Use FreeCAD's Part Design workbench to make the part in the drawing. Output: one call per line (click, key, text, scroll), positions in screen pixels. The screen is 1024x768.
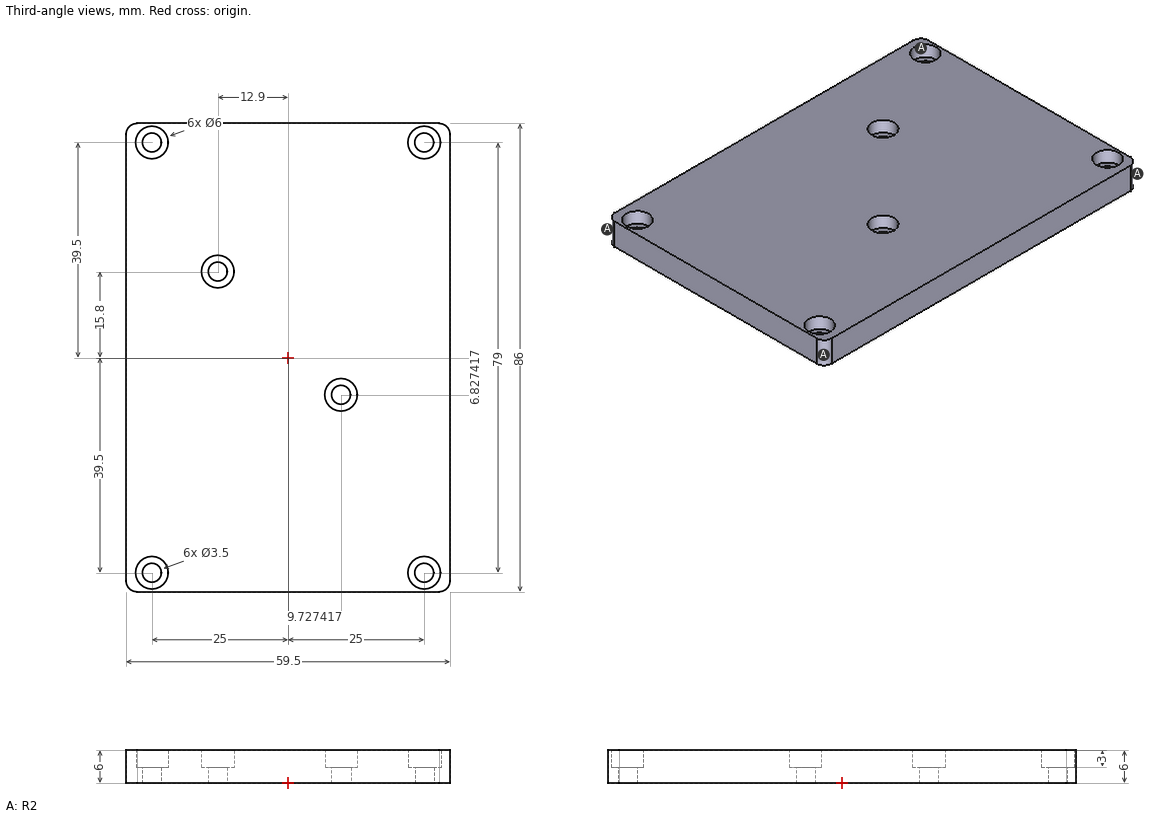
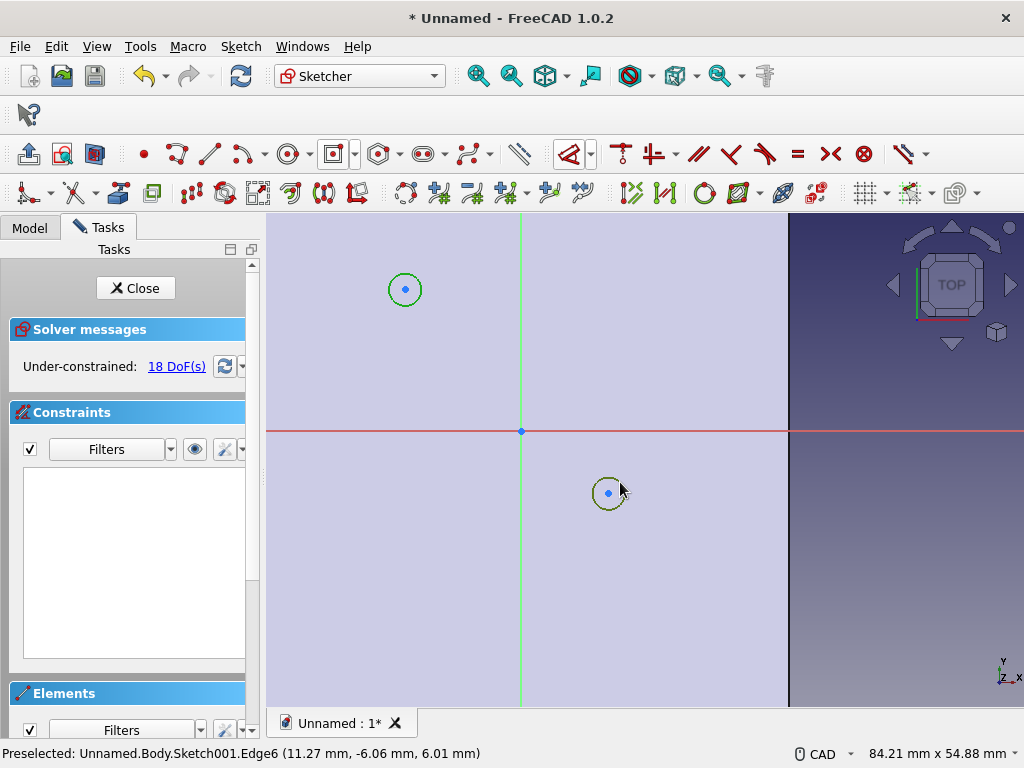
key(e)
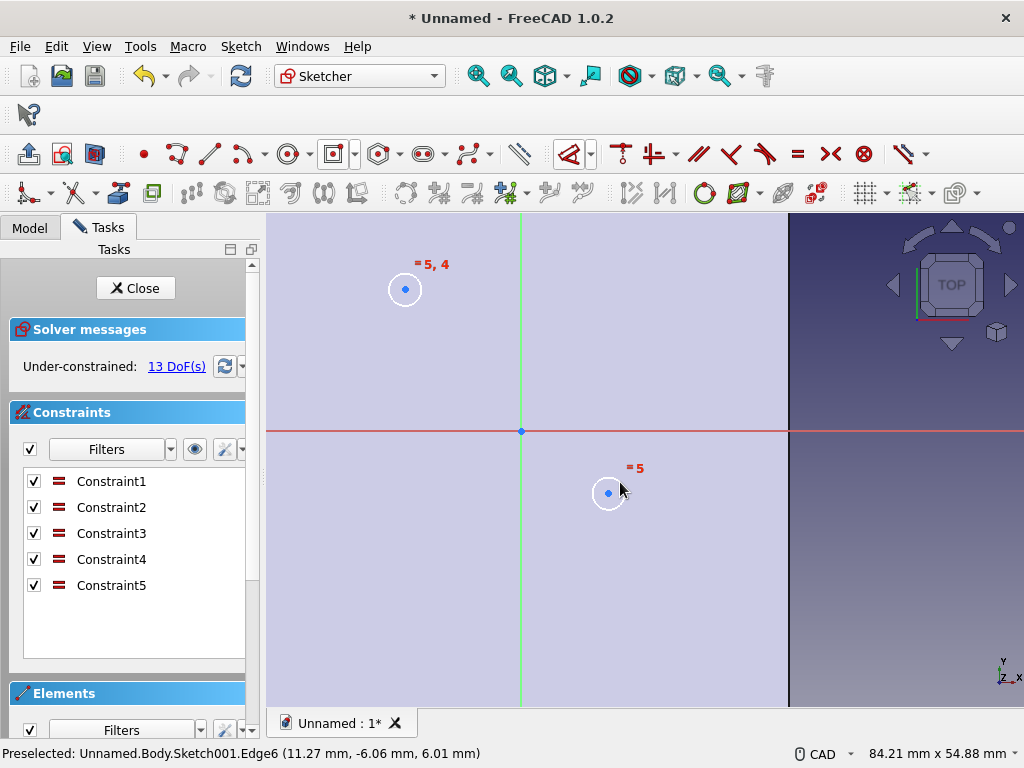
scroll(621, 483, down, 4)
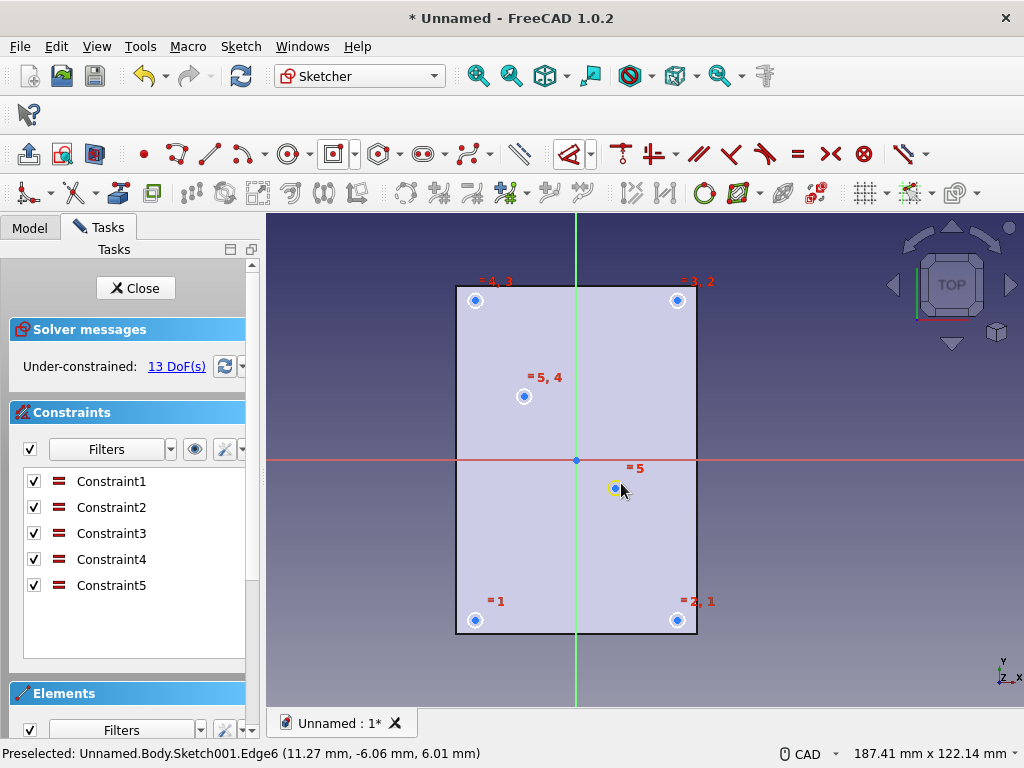
click(475, 620)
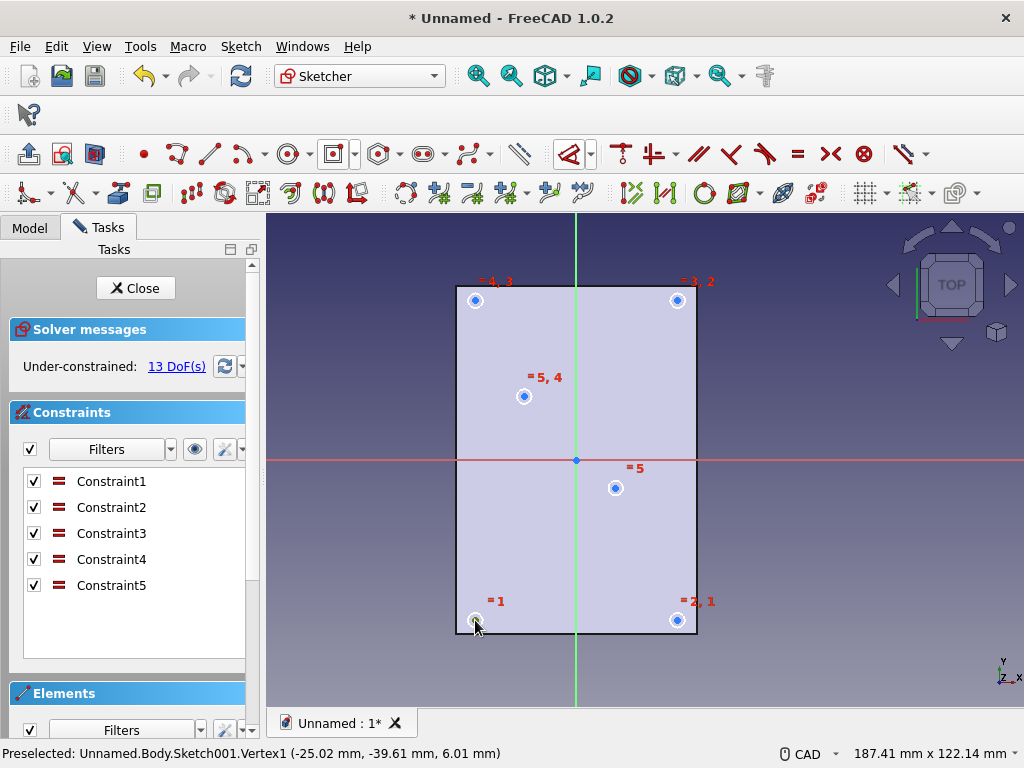
click(677, 620)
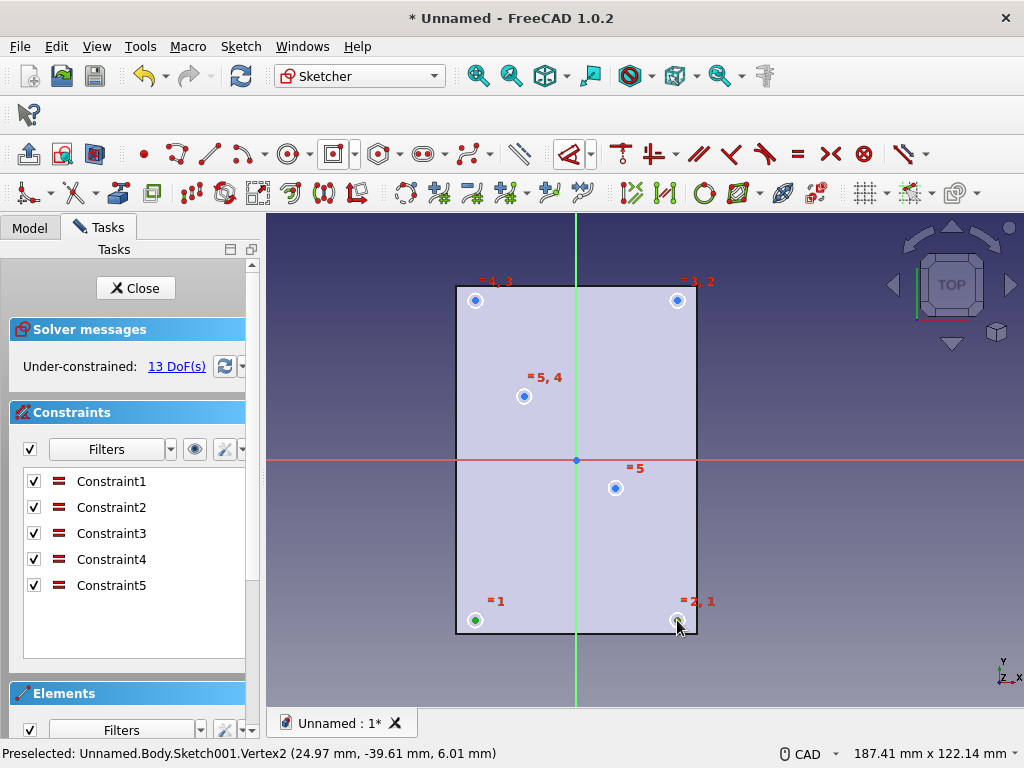
key(h)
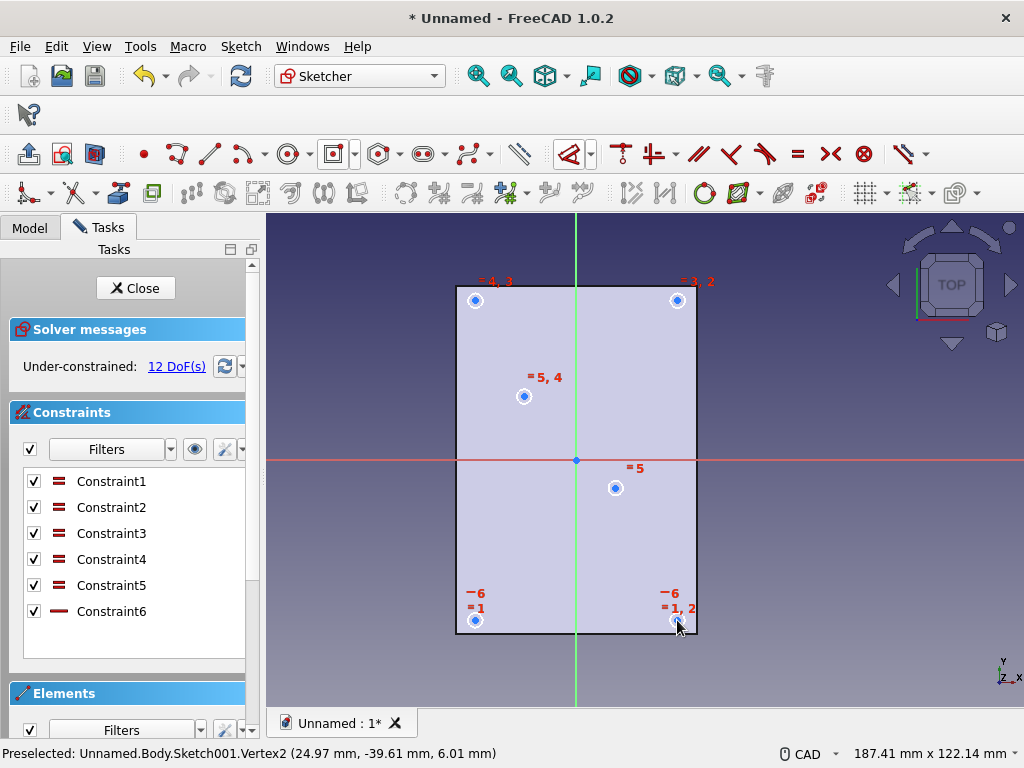
click(677, 620)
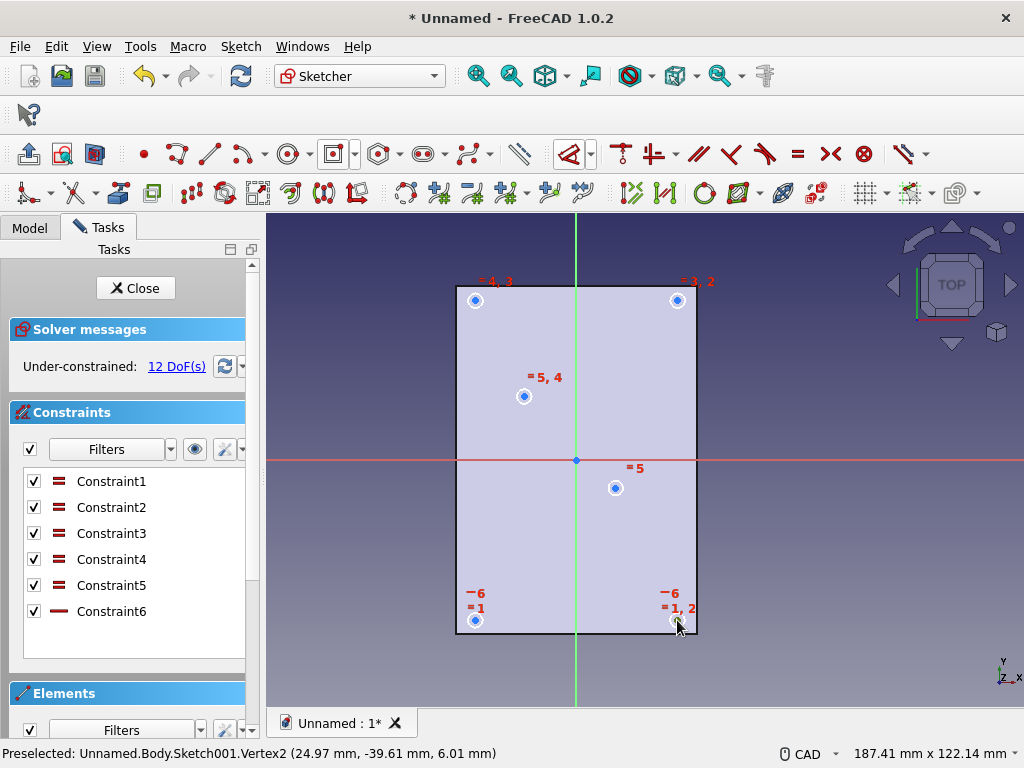
click(678, 301)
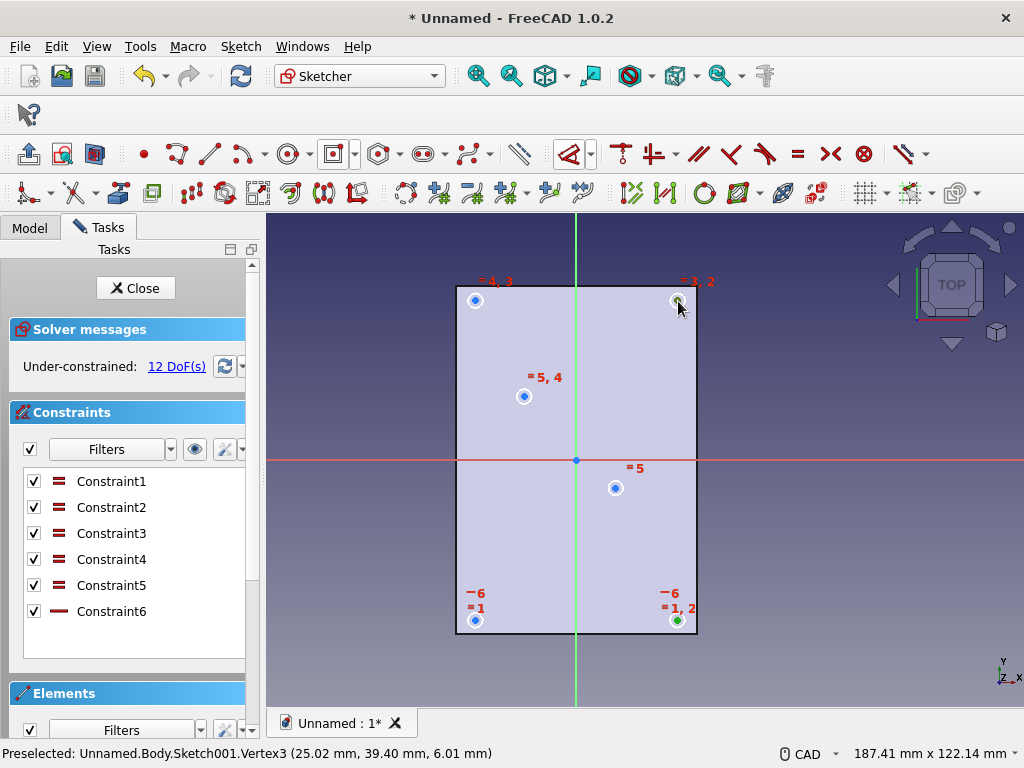
key(v)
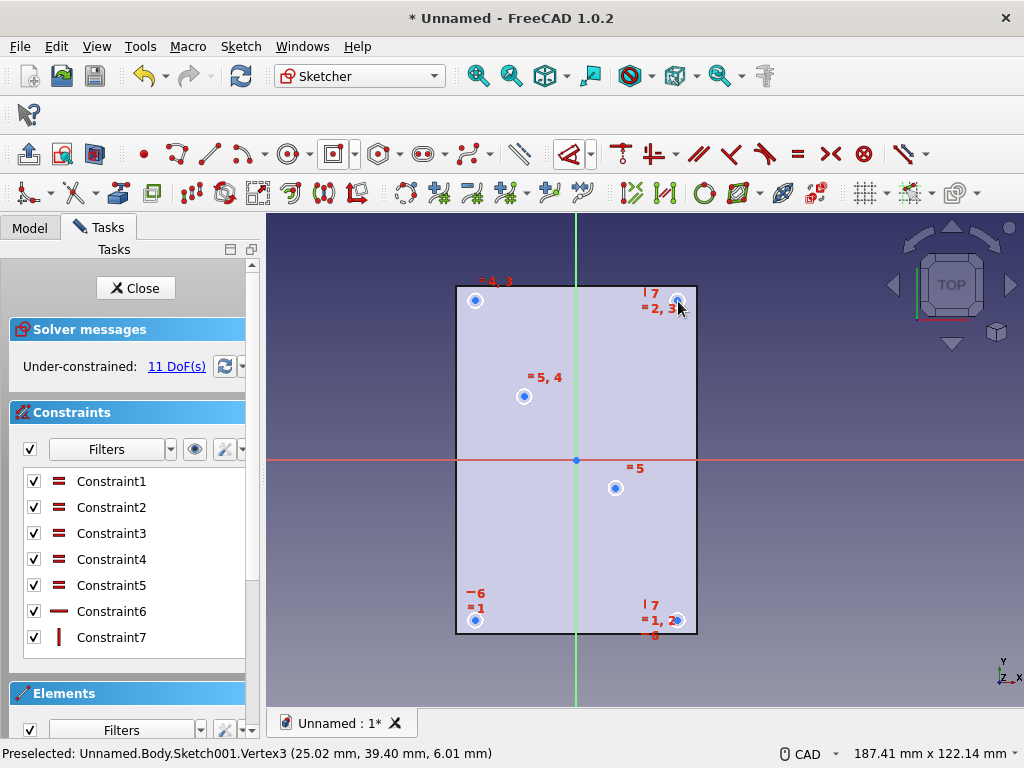
click(475, 620)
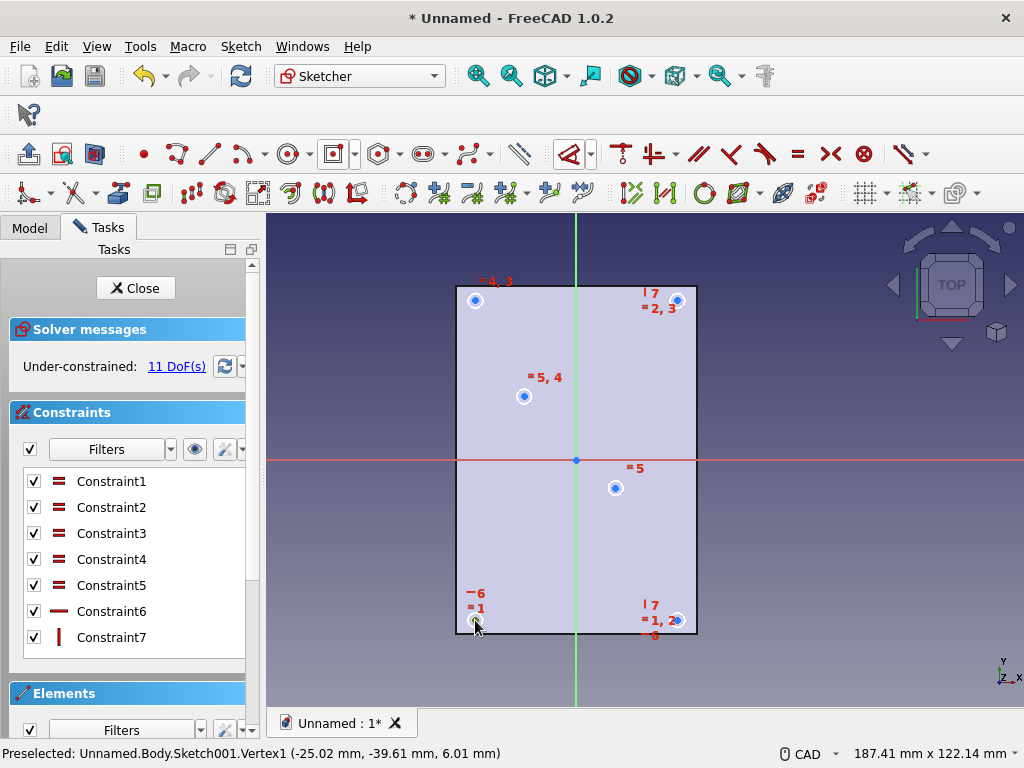
click(475, 301)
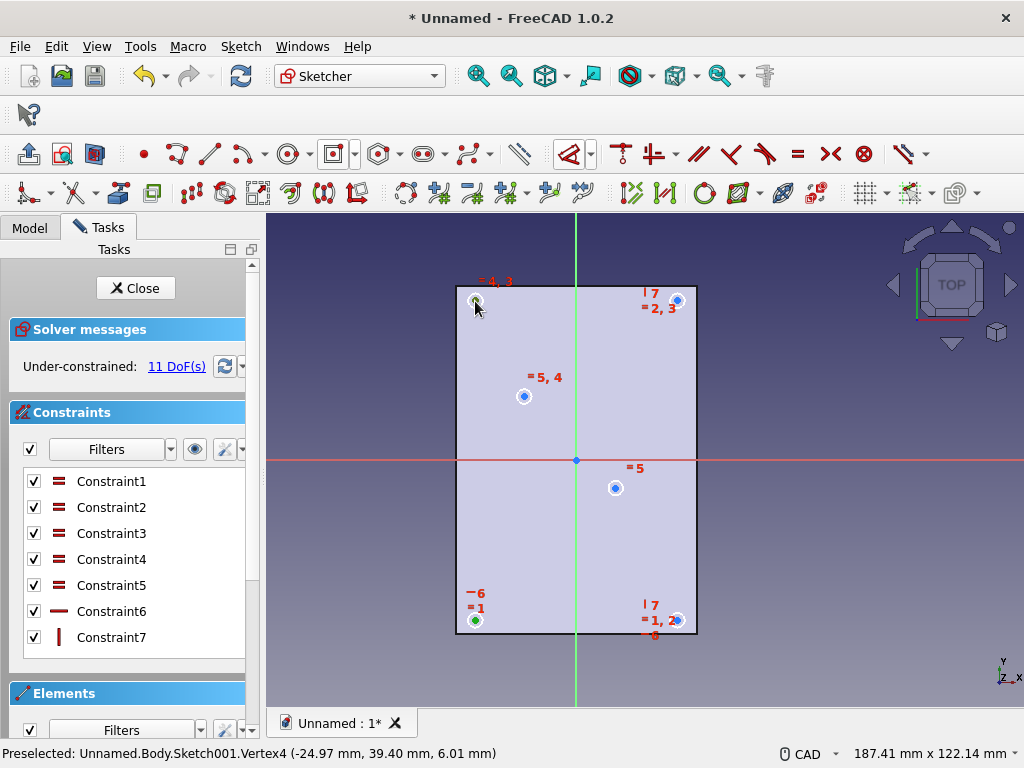
key(v)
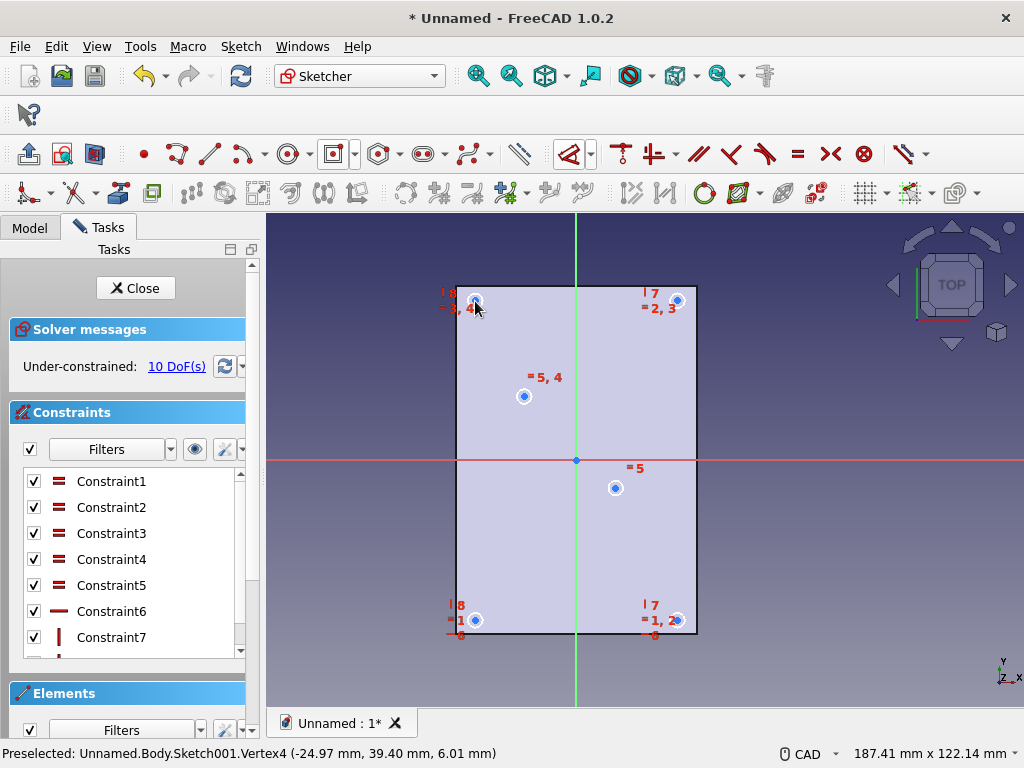
click(677, 301)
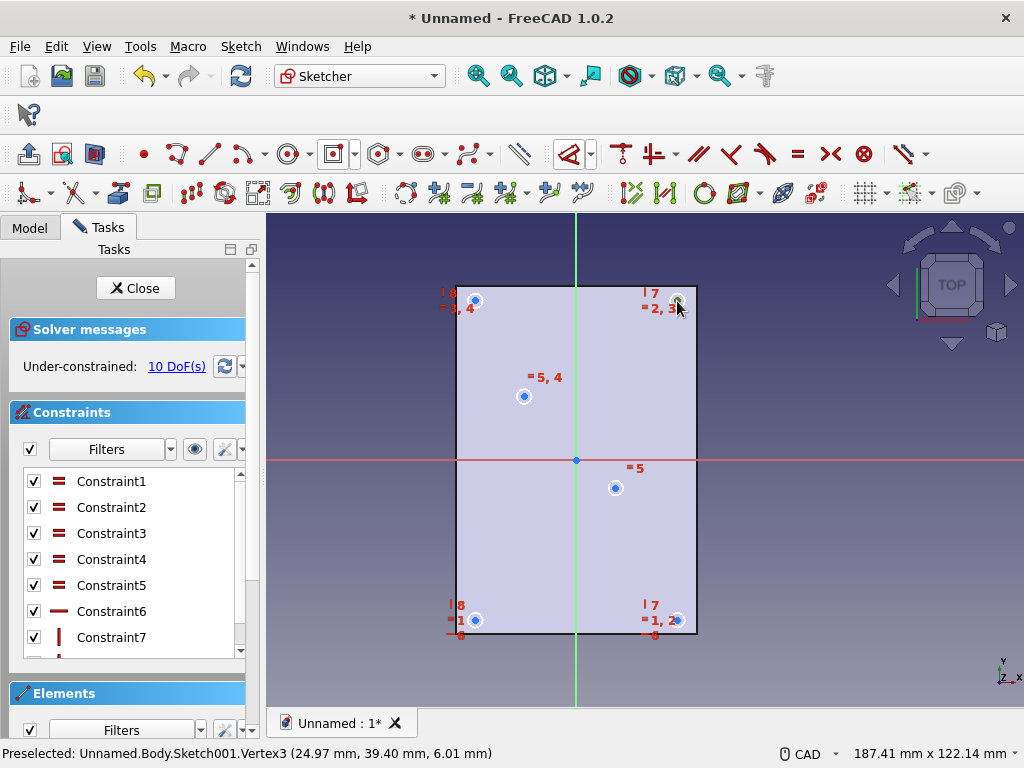
click(475, 301)